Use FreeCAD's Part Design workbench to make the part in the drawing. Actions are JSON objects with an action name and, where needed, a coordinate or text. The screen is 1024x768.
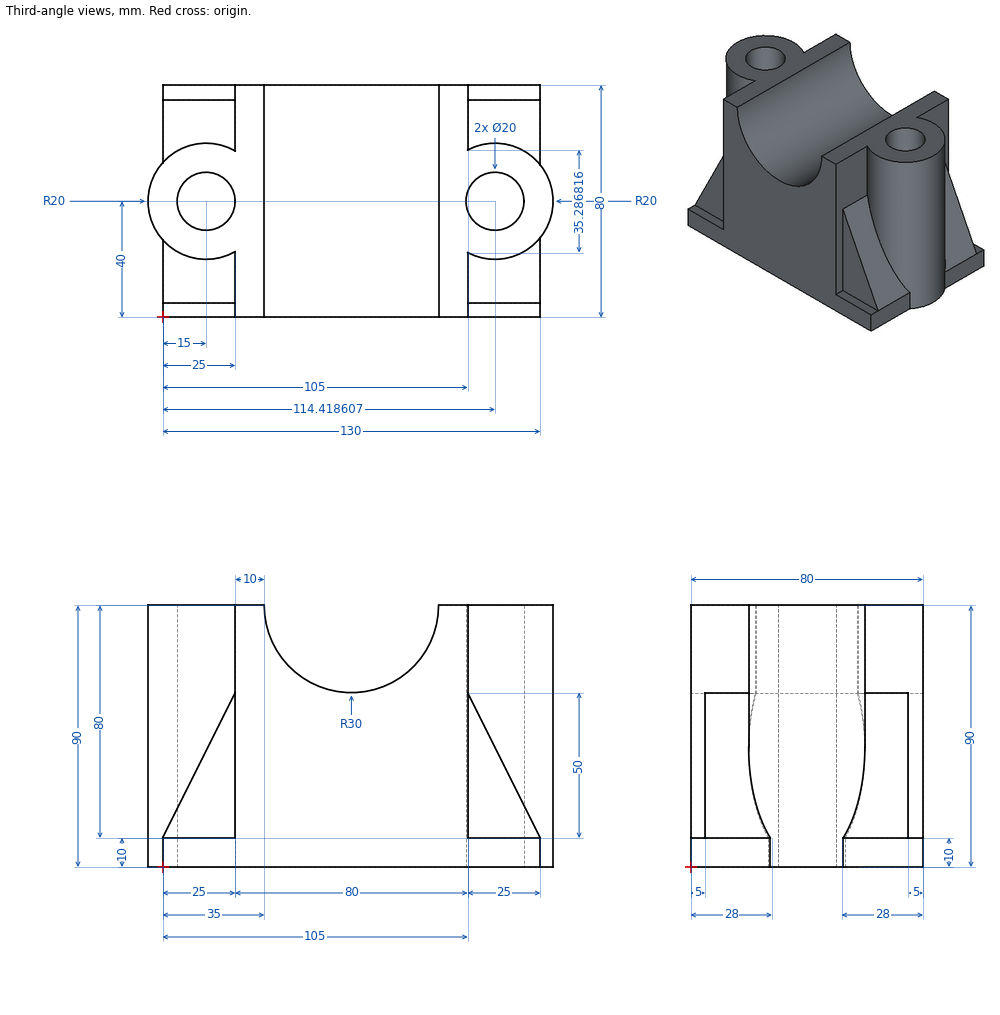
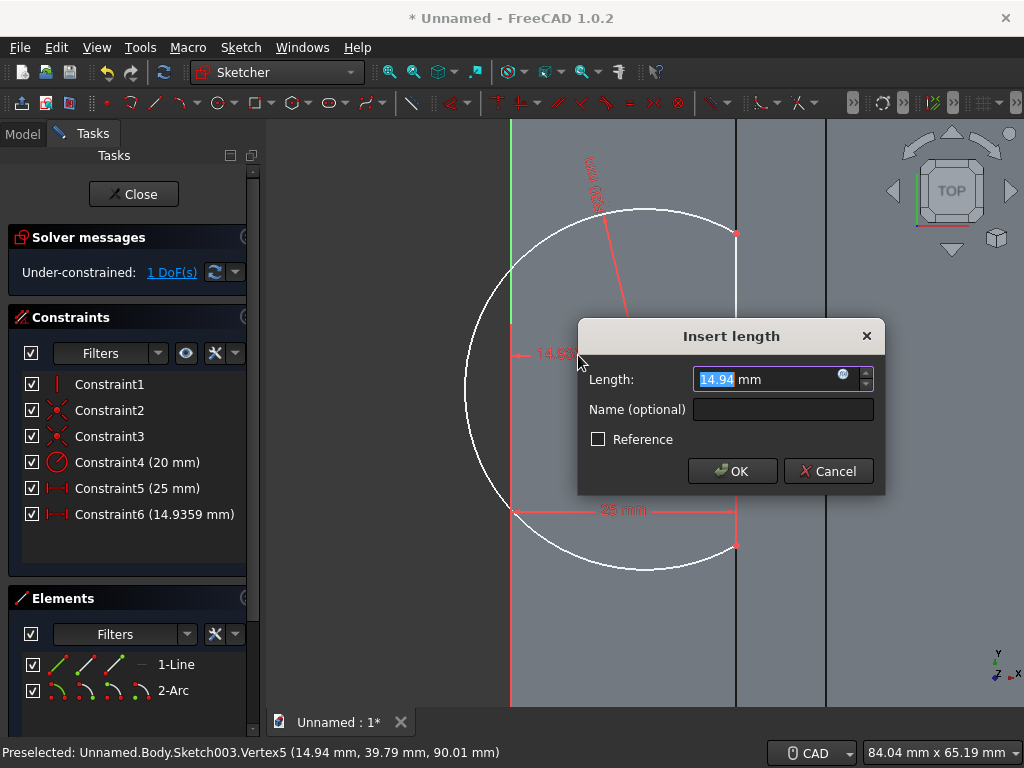
{"action": "type", "text": "15"}
{"action": "key", "text": "Return"}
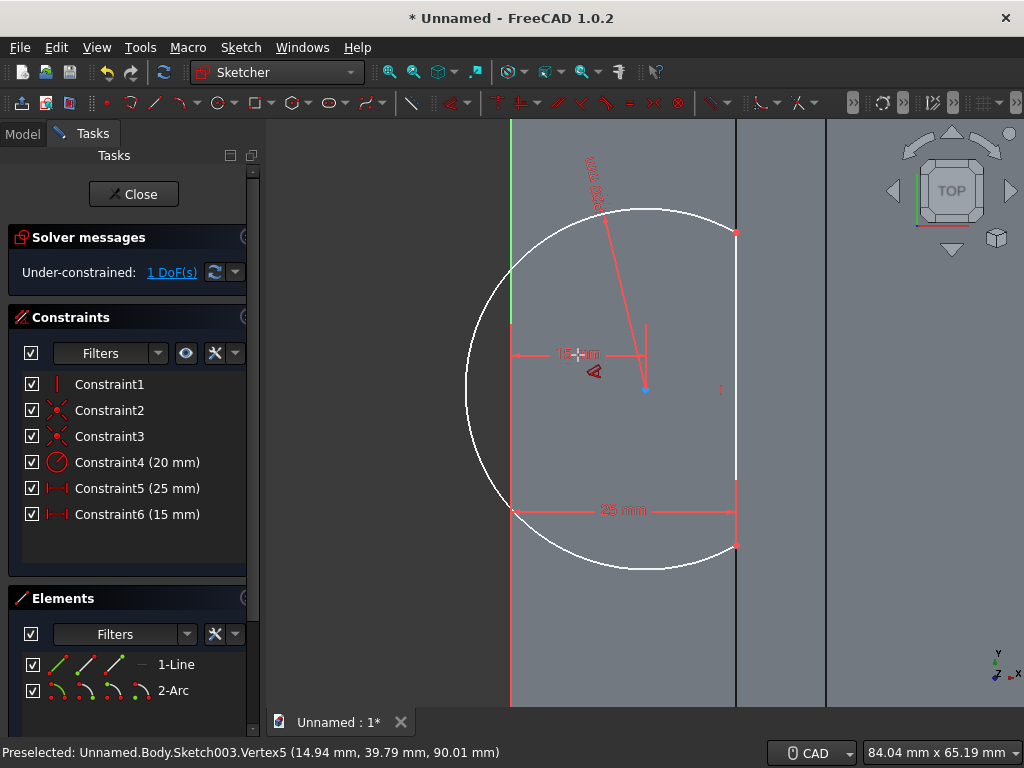
{"action": "left_click", "coordinate": [646, 389]}
{"action": "left_click", "coordinate": [477, 534]}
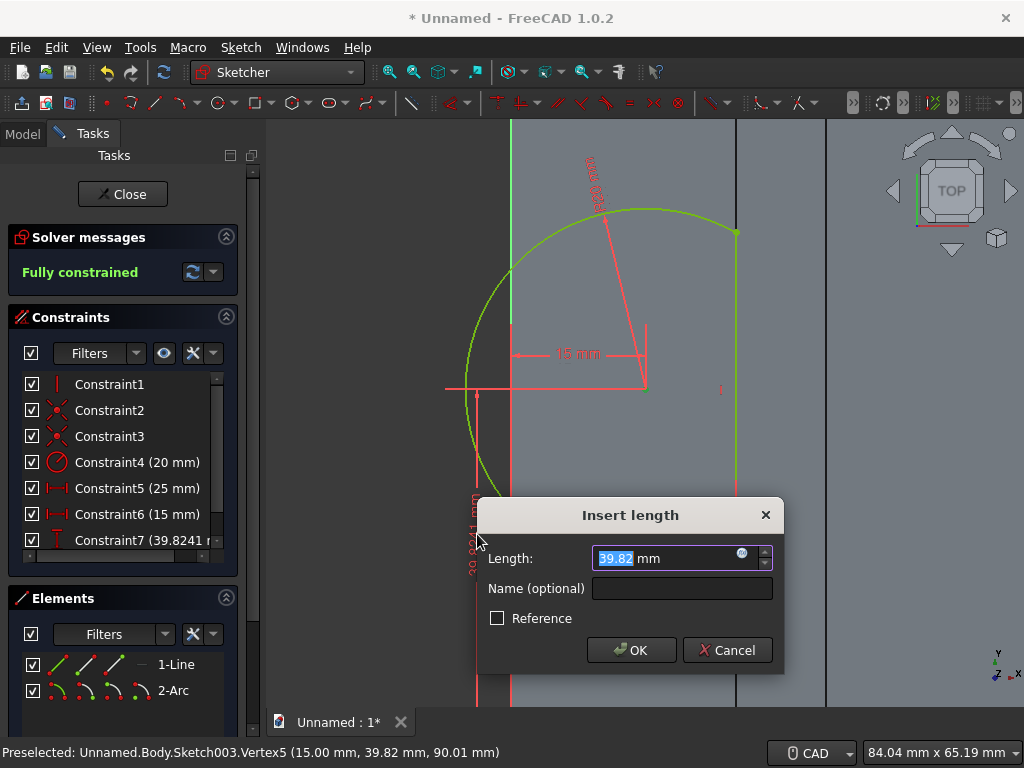
{"action": "type", "text": "40"}
{"action": "key", "text": "Return"}
{"action": "key", "text": "Escape"}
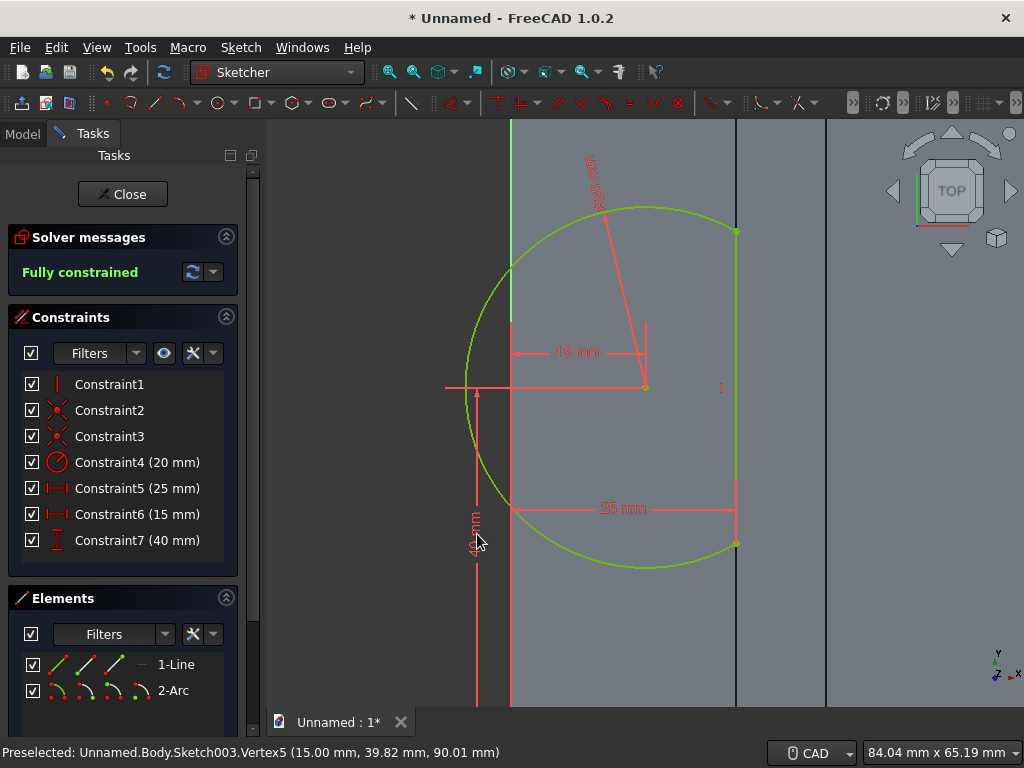
{"action": "left_click", "coordinate": [123, 194]}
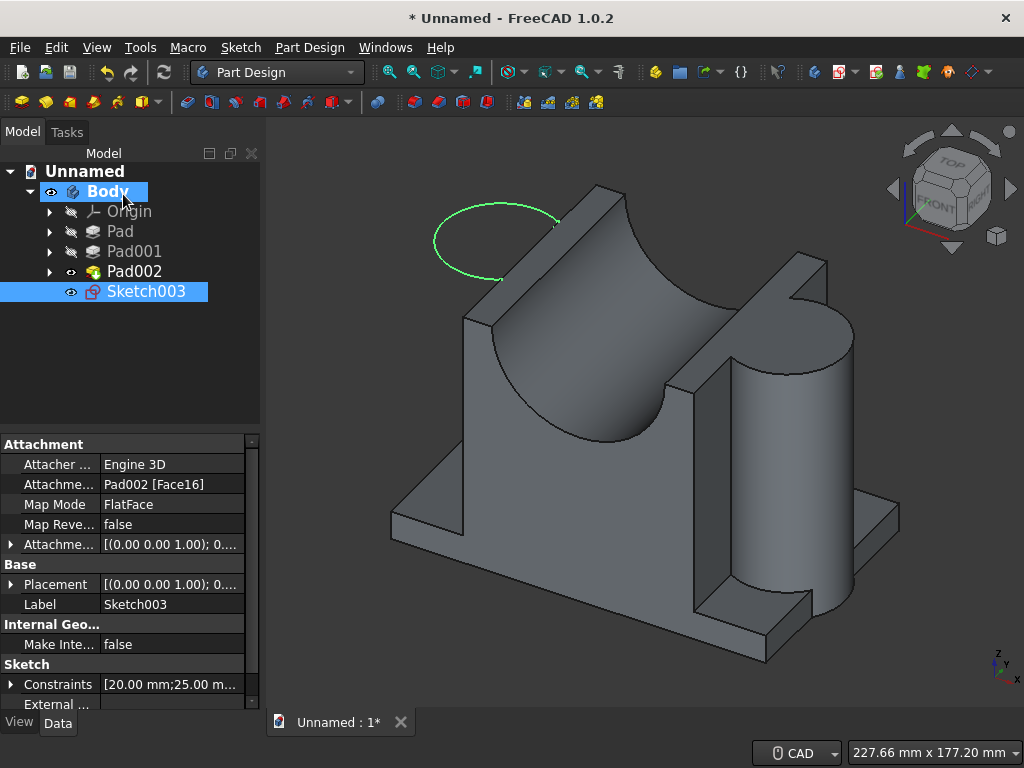
{"action": "left_click", "coordinate": [22, 102]}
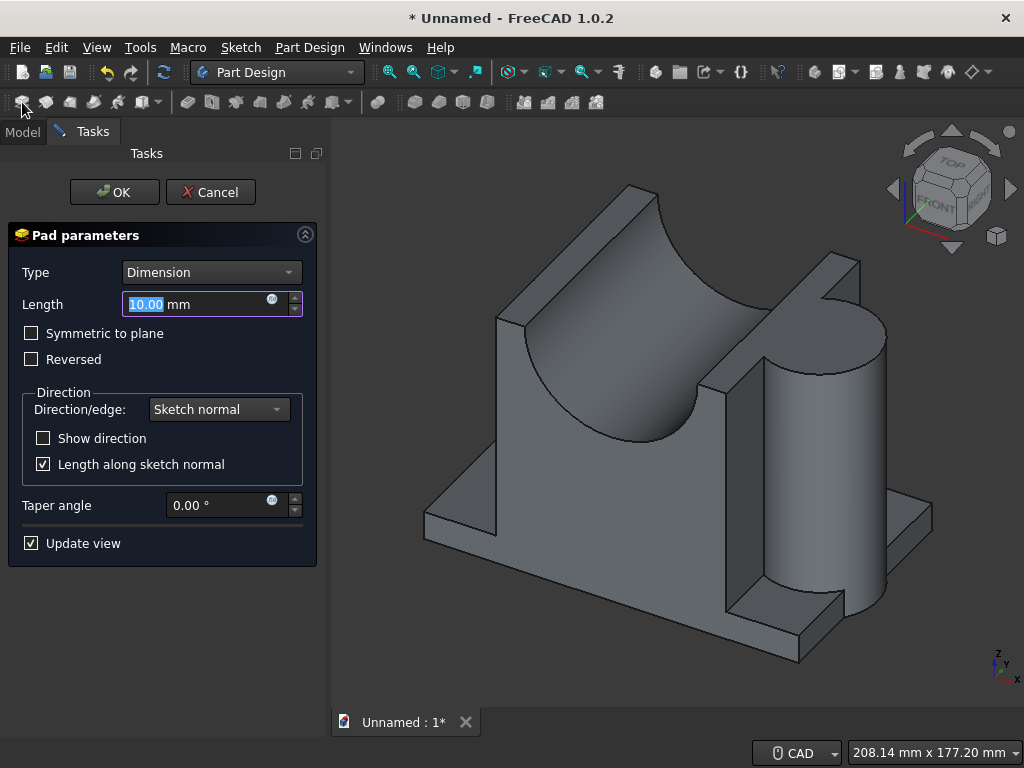
{"action": "type", "text": "90"}
{"action": "key", "text": "Tab"}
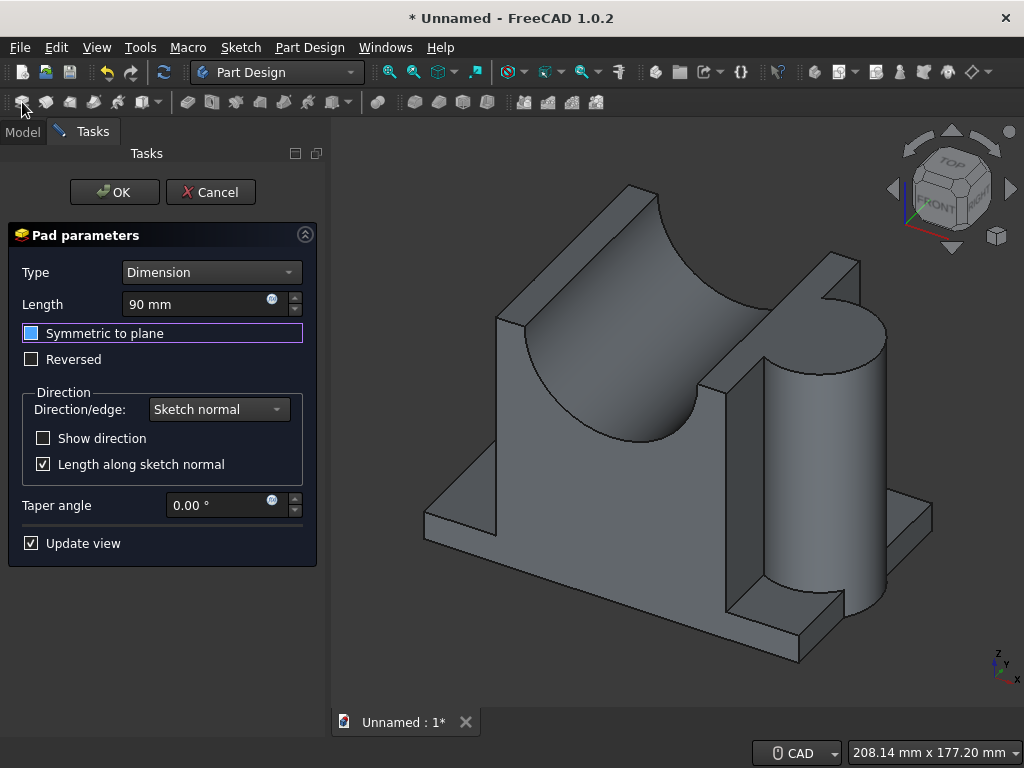
{"action": "left_click", "coordinate": [30, 359]}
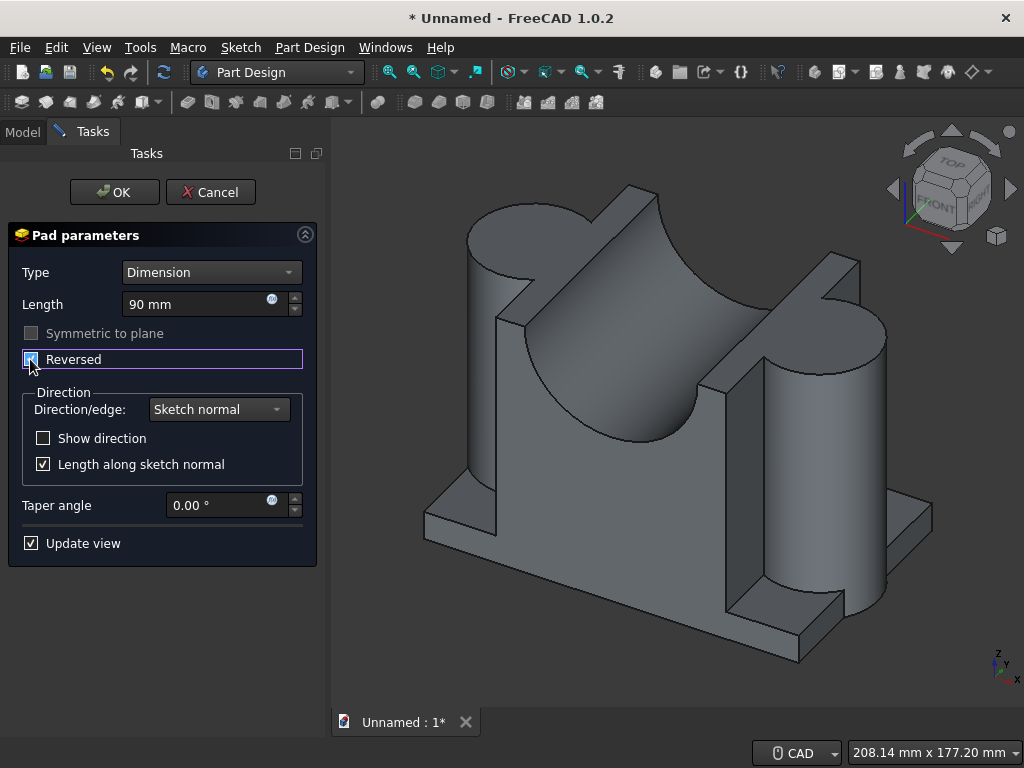
{"action": "left_click", "coordinate": [115, 192]}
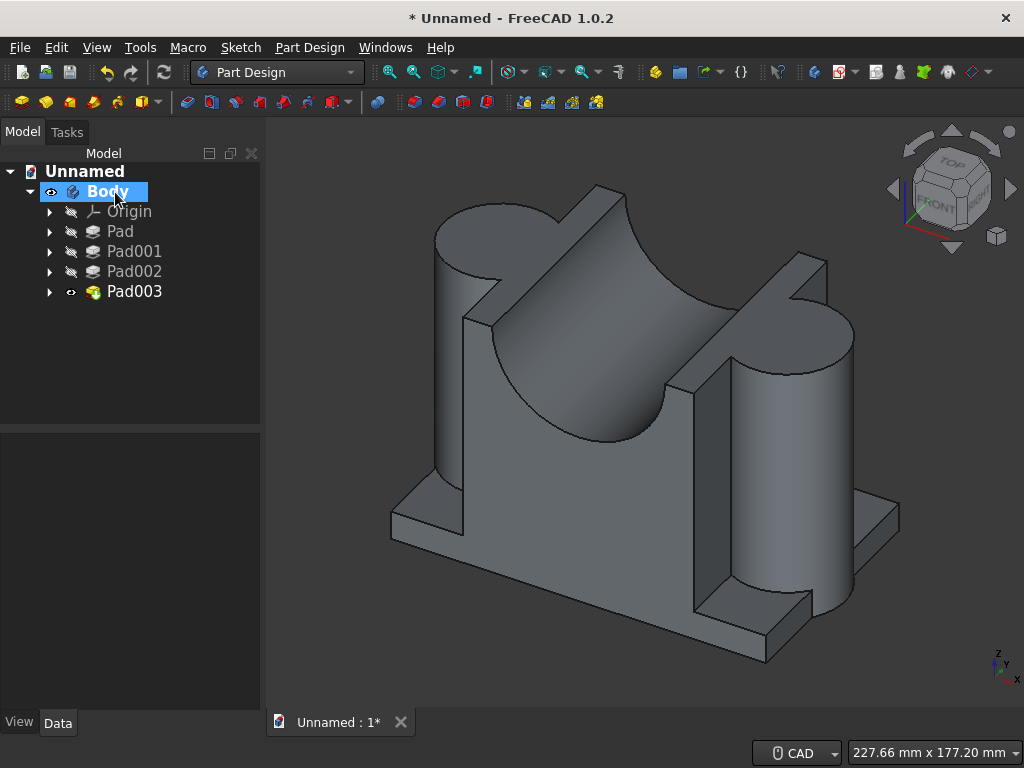
{"action": "left_click", "coordinate": [501, 241]}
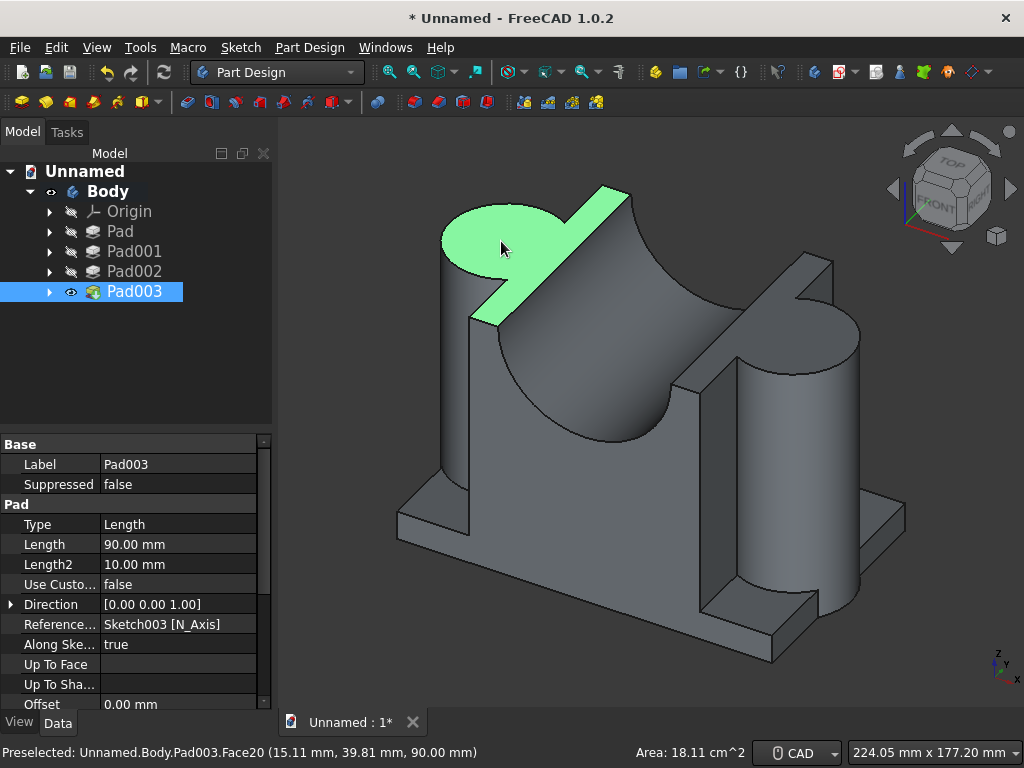
{"action": "left_click", "coordinate": [840, 72]}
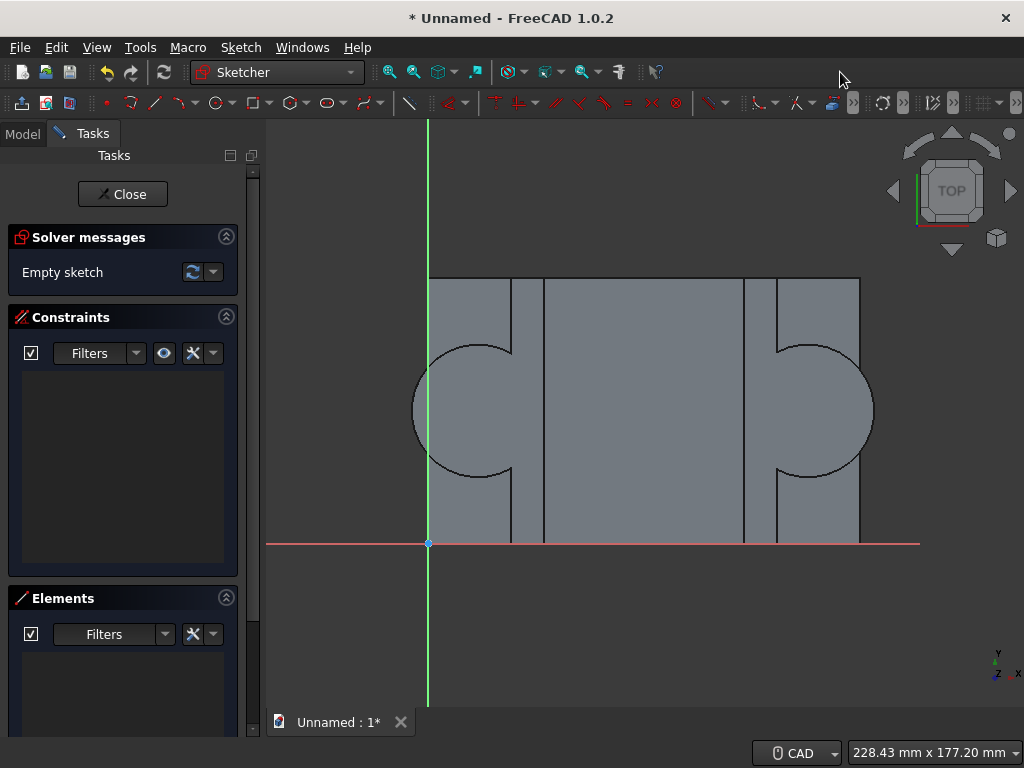
{"action": "scroll", "coordinate": [313, 198], "scroll_direction": "down", "scroll_amount": 1}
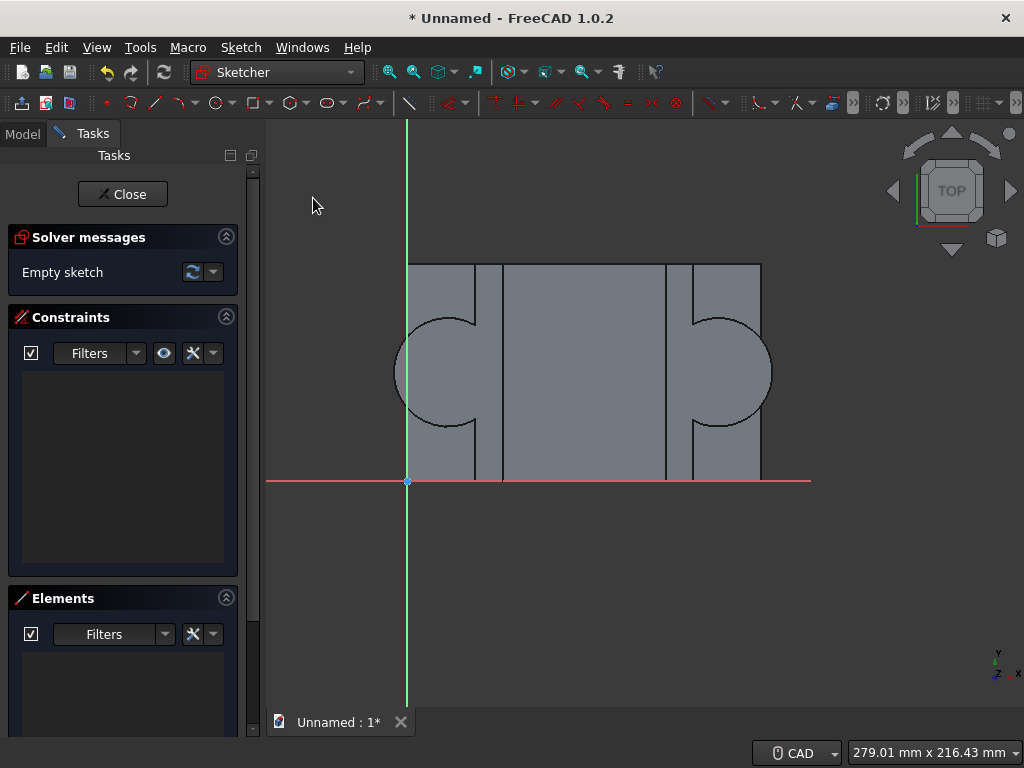
{"action": "left_click", "coordinate": [216, 104]}